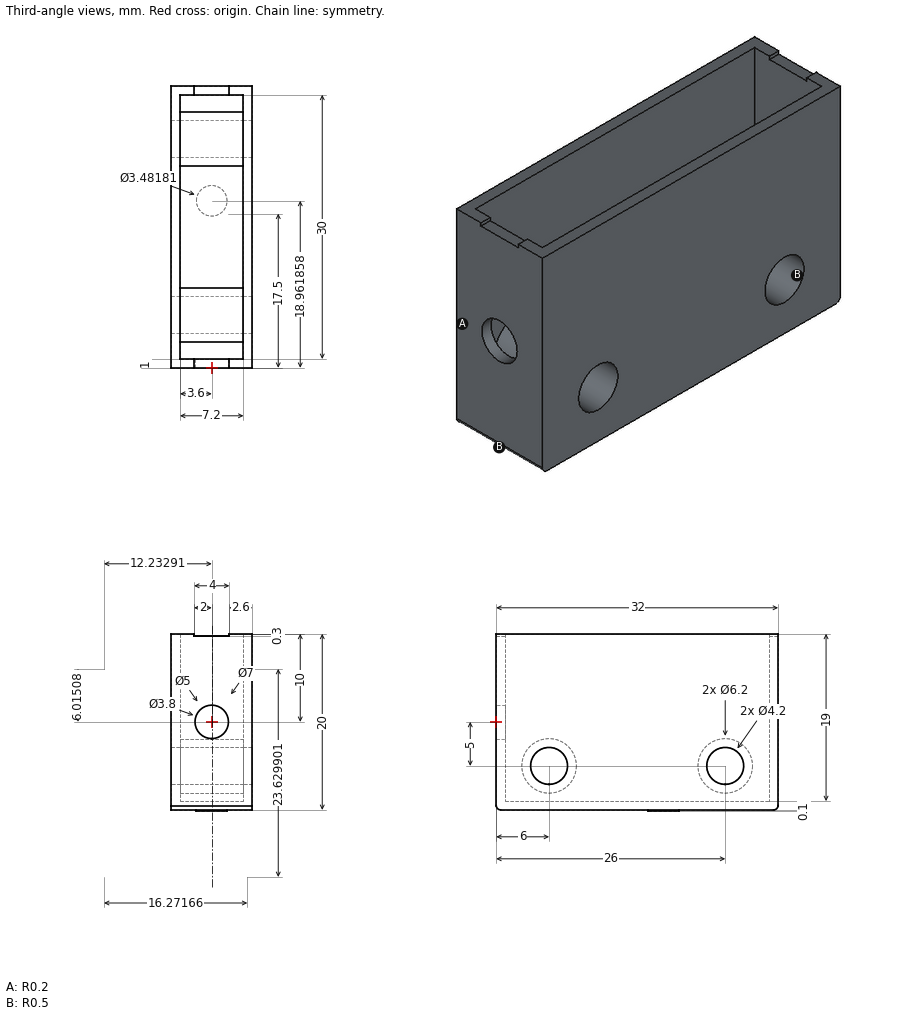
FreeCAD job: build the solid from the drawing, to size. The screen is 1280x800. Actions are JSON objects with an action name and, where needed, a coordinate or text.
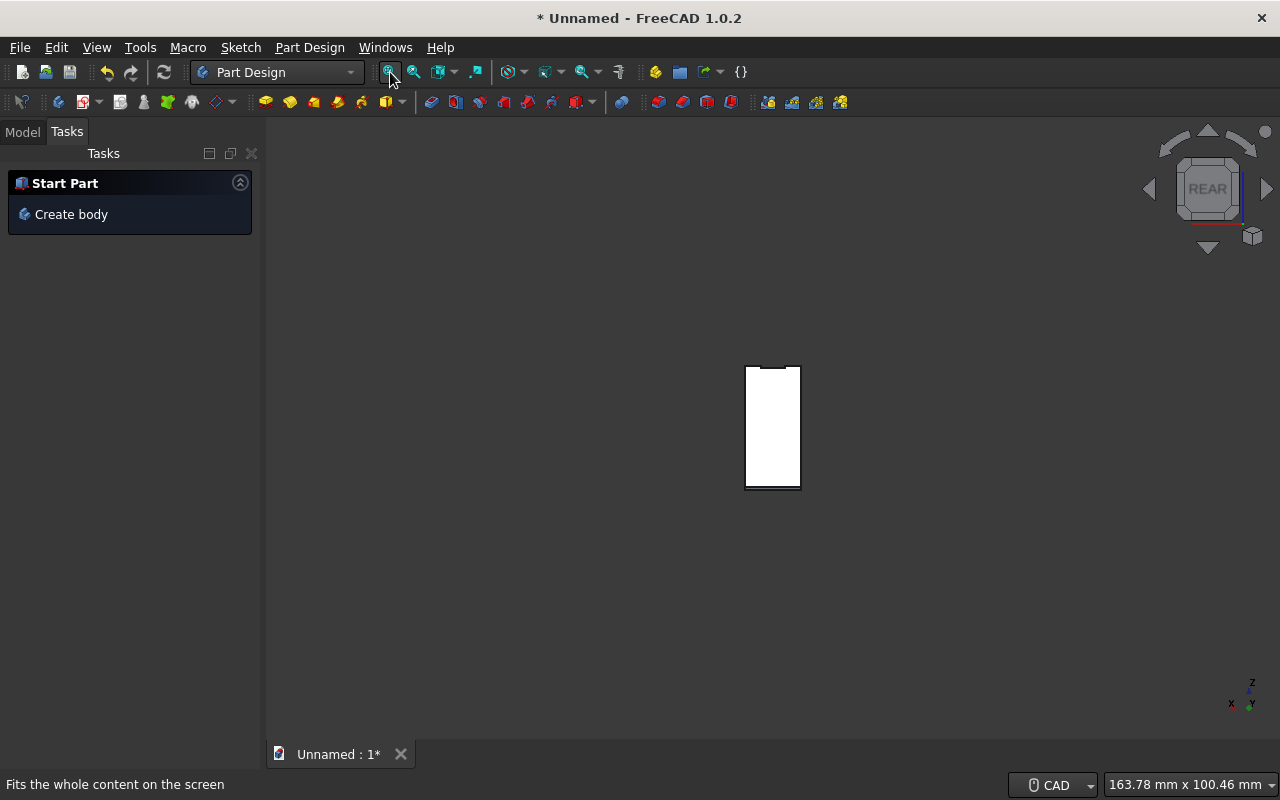
{"action": "key", "text": "0"}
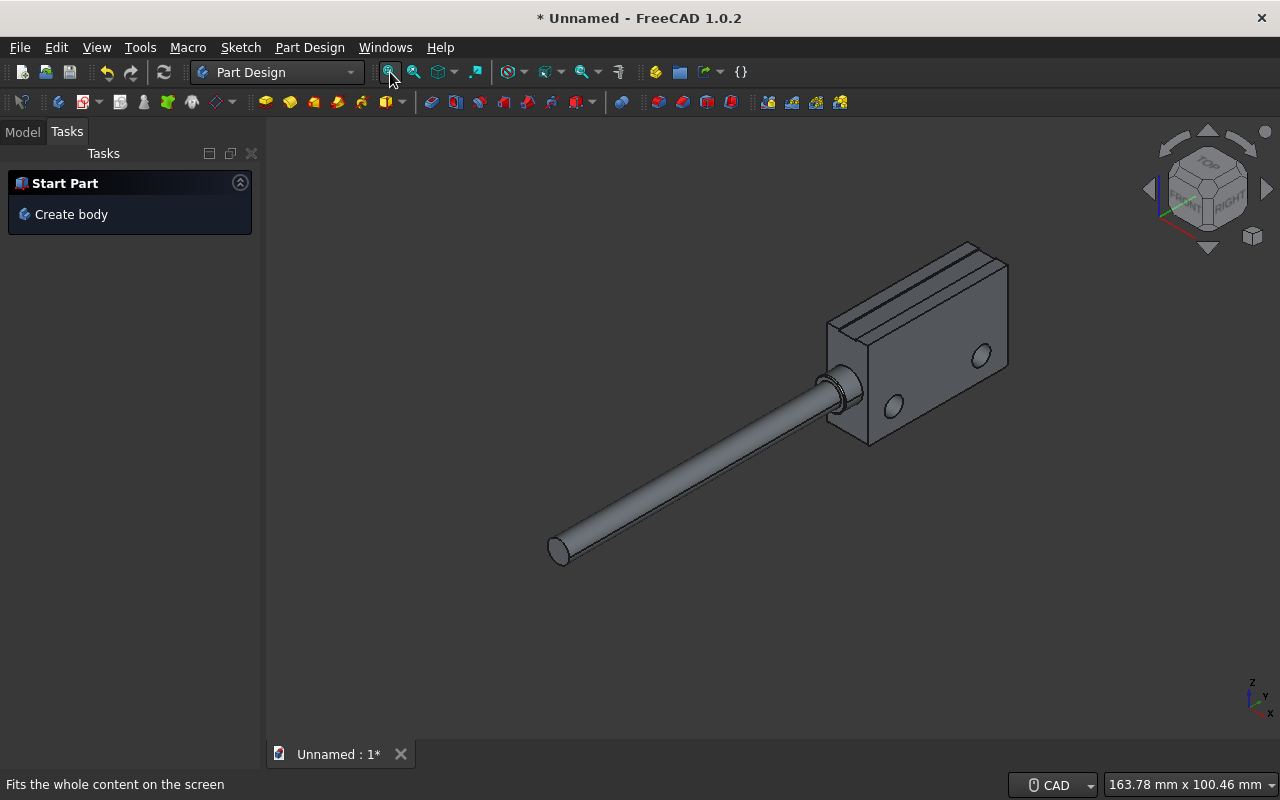
{"action": "key", "text": "2"}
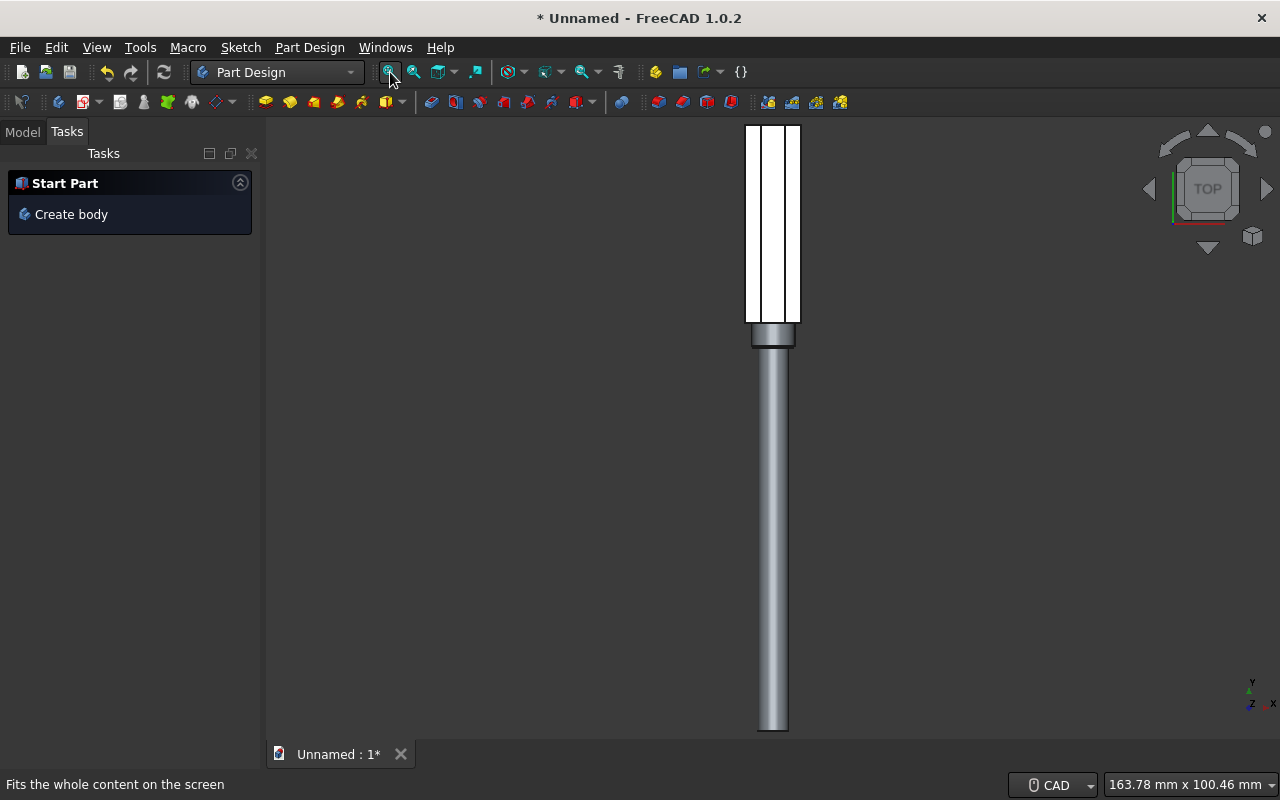
{"action": "key", "text": "4"}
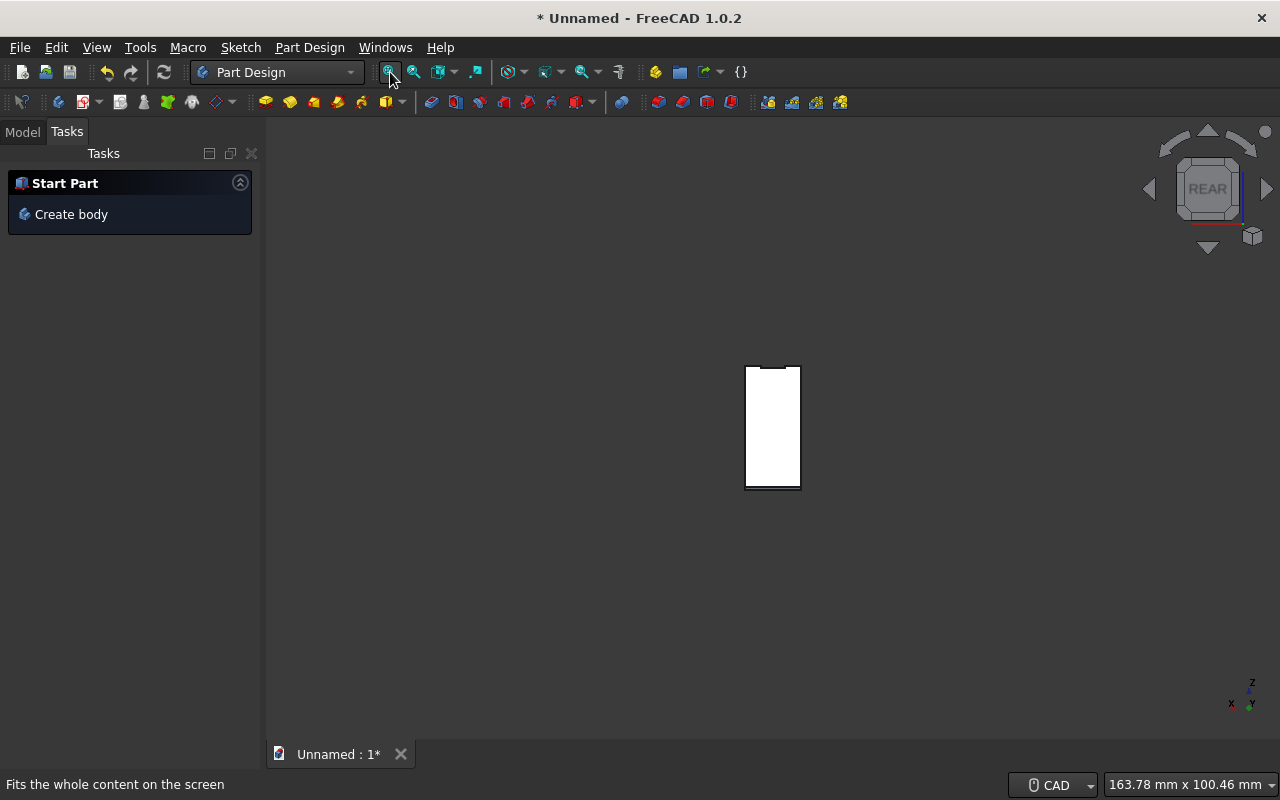
{"action": "left_click", "coordinate": [390, 72]}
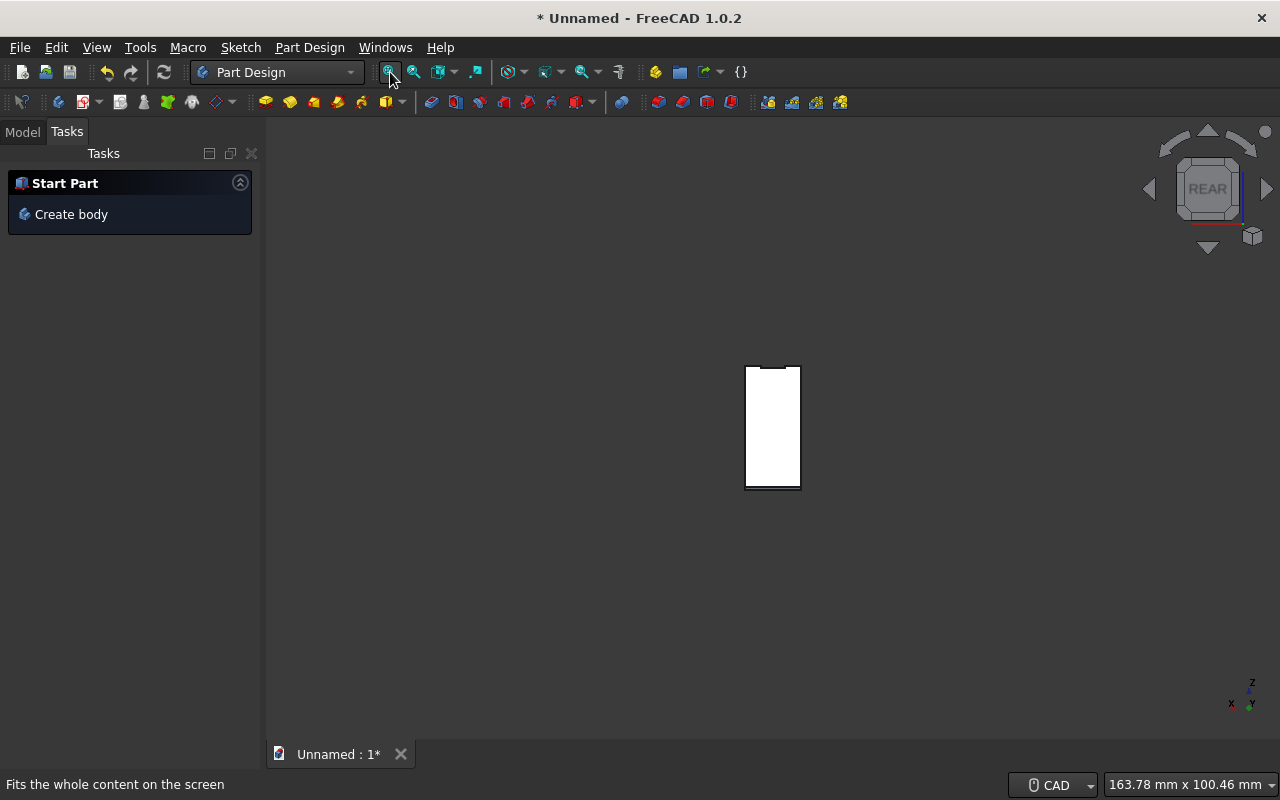
{"action": "left_click", "coordinate": [23, 131]}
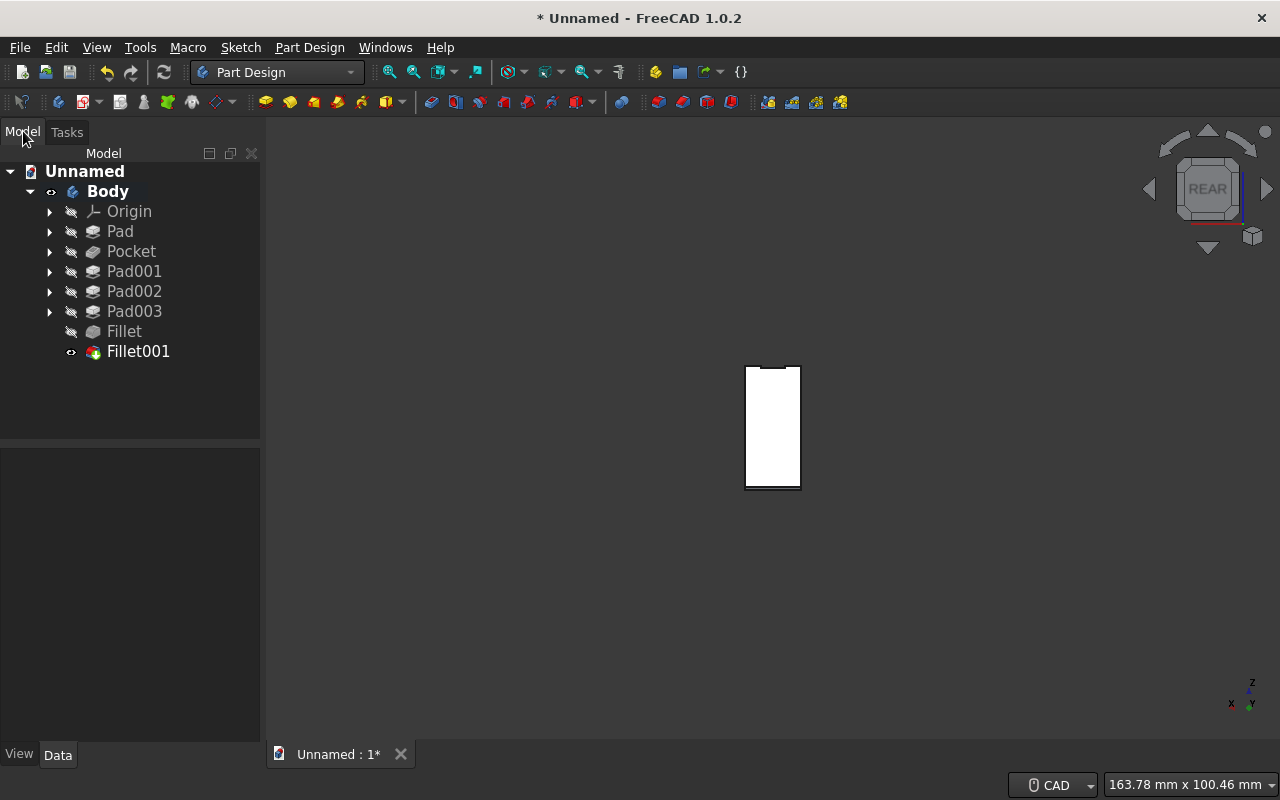
{"action": "left_click", "coordinate": [50, 212]}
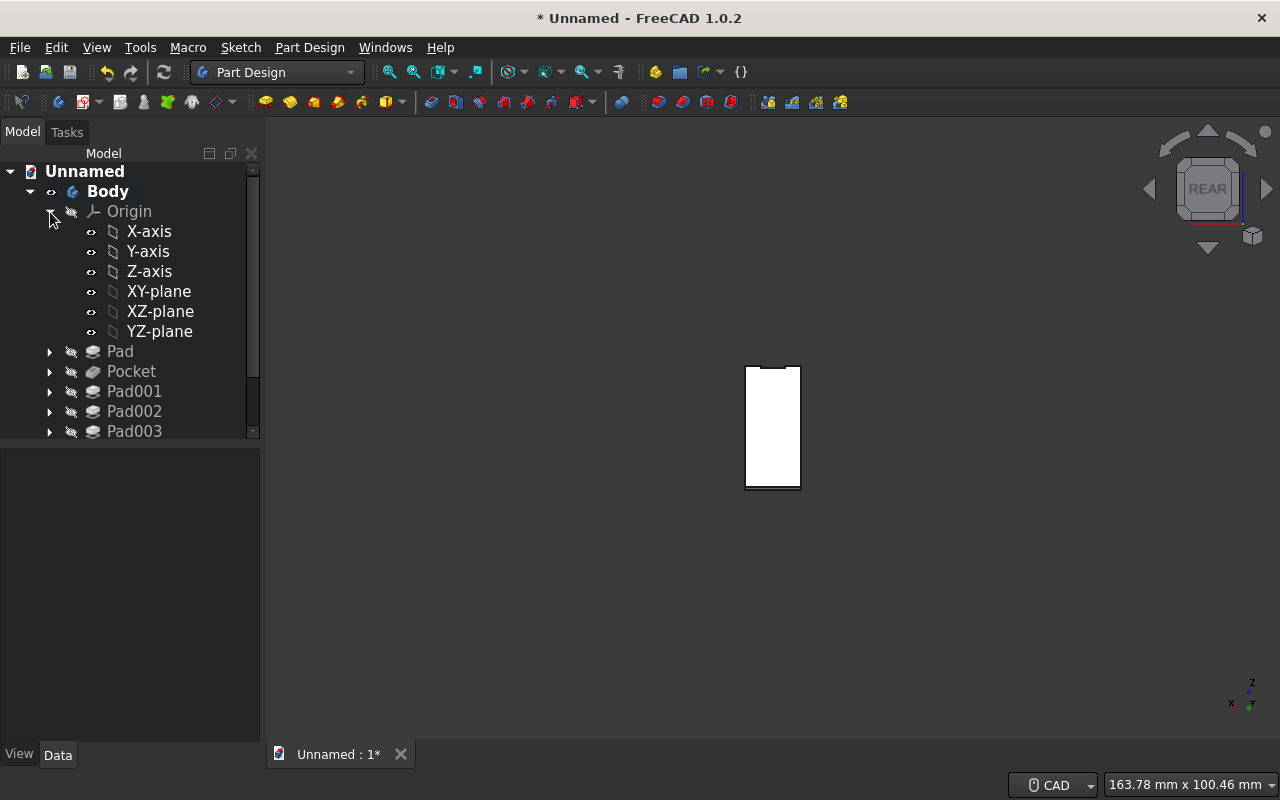
{"action": "left_click", "coordinate": [136, 292]}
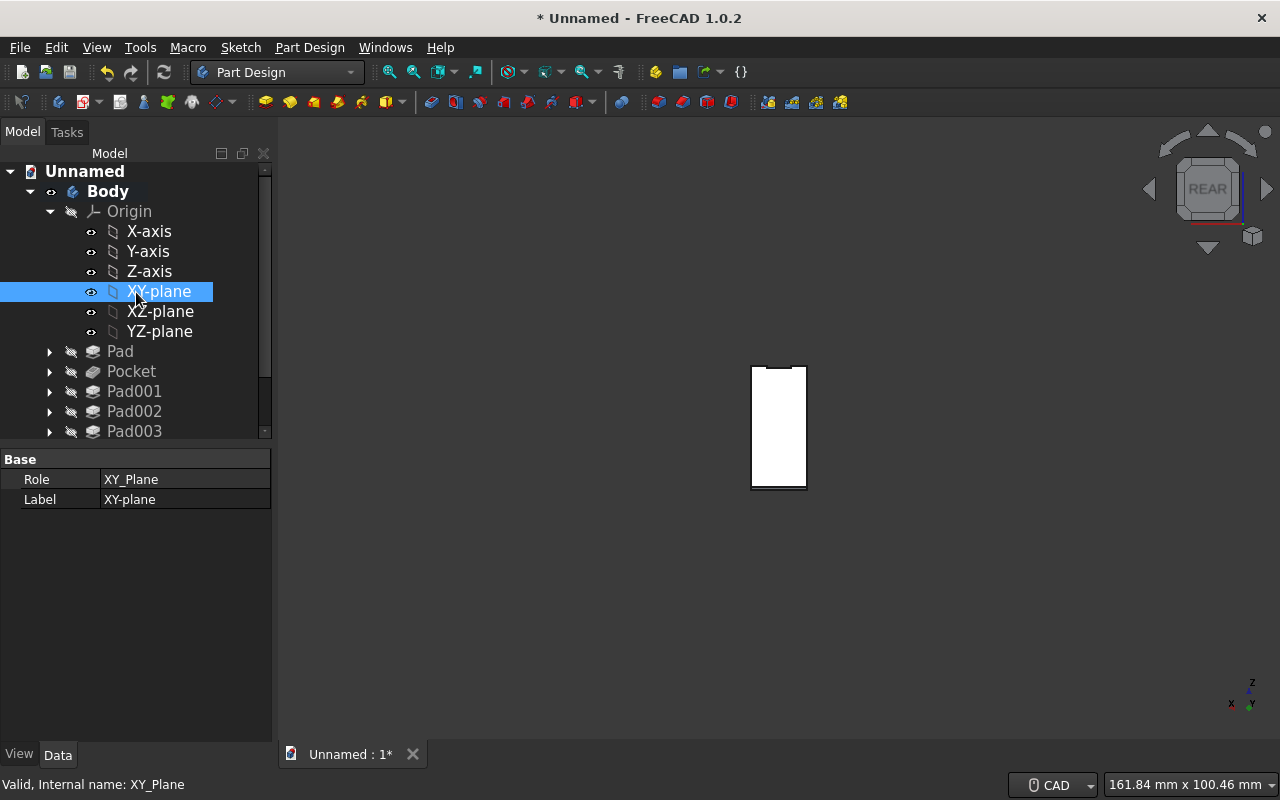
{"action": "left_click", "coordinate": [216, 102]}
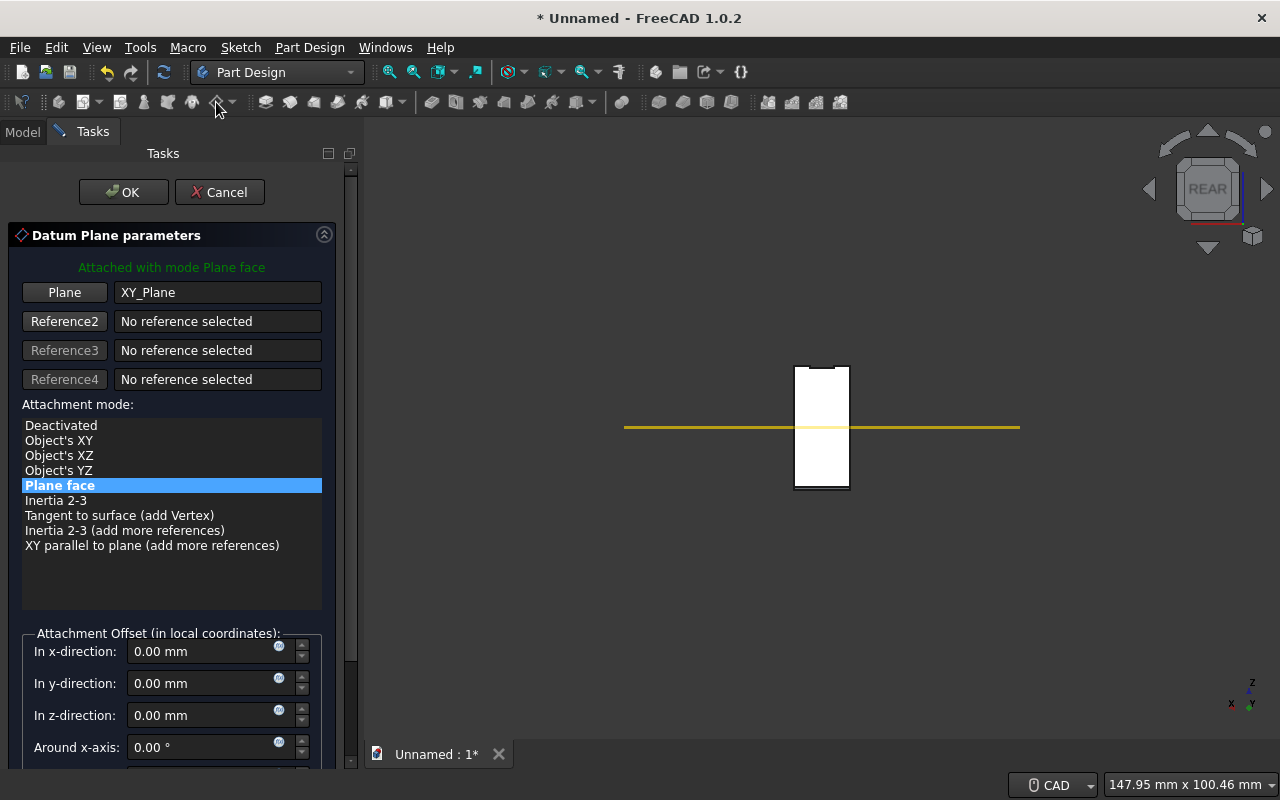
{"action": "triple_click", "coordinate": [210, 715]}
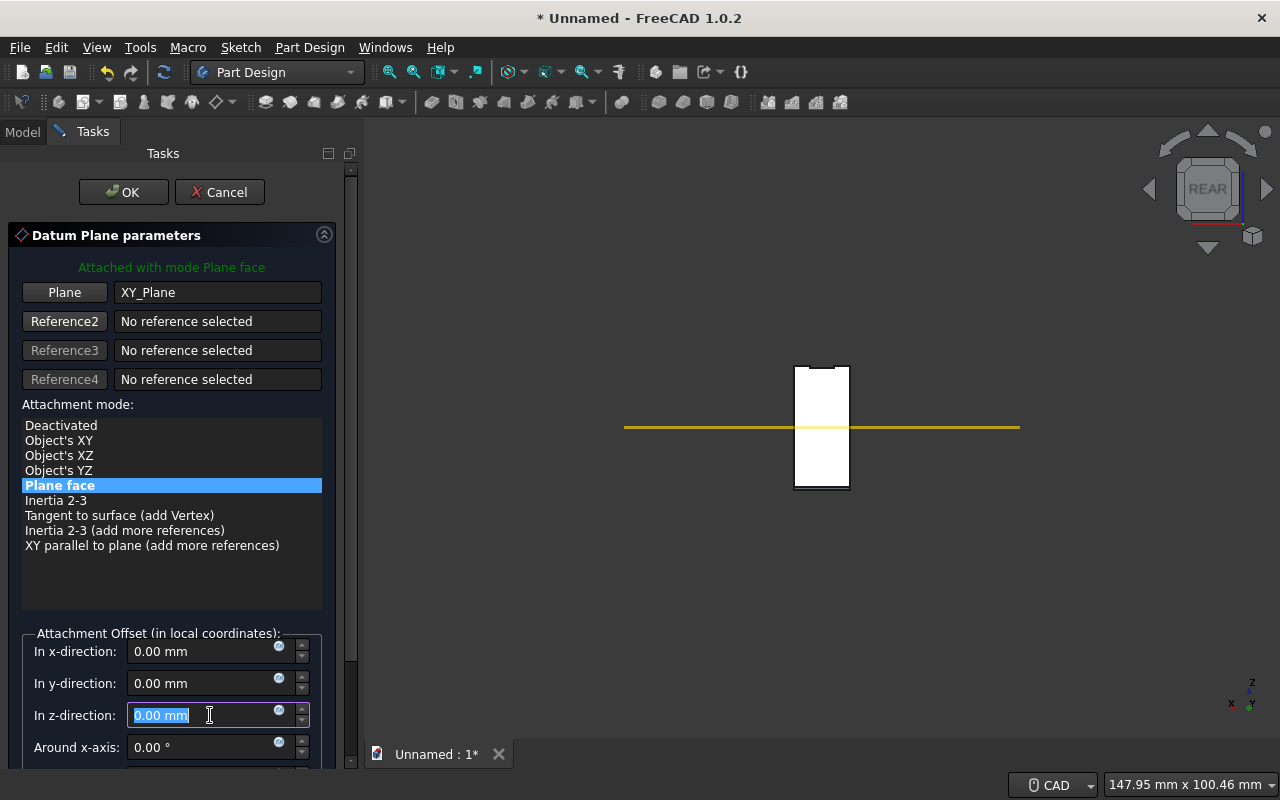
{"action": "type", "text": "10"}
{"action": "key", "text": "Tab"}